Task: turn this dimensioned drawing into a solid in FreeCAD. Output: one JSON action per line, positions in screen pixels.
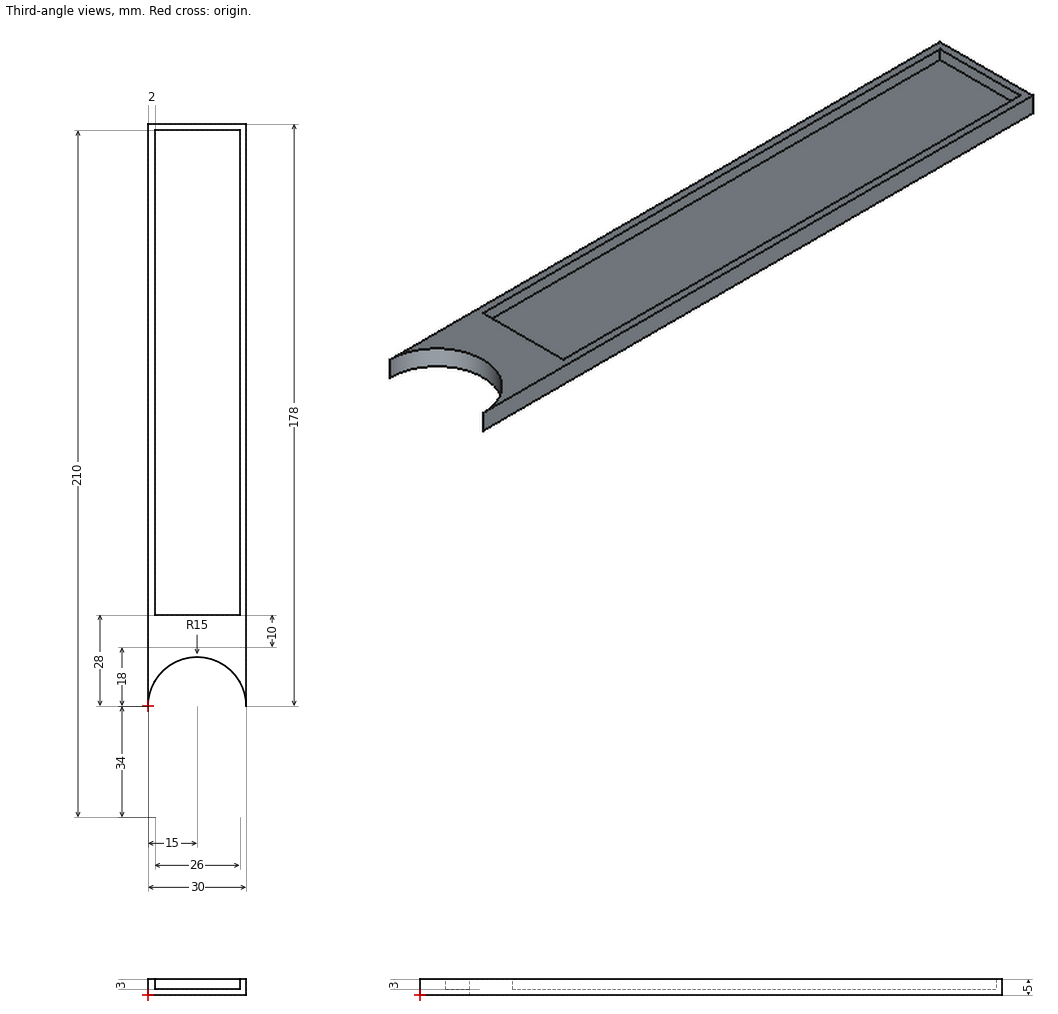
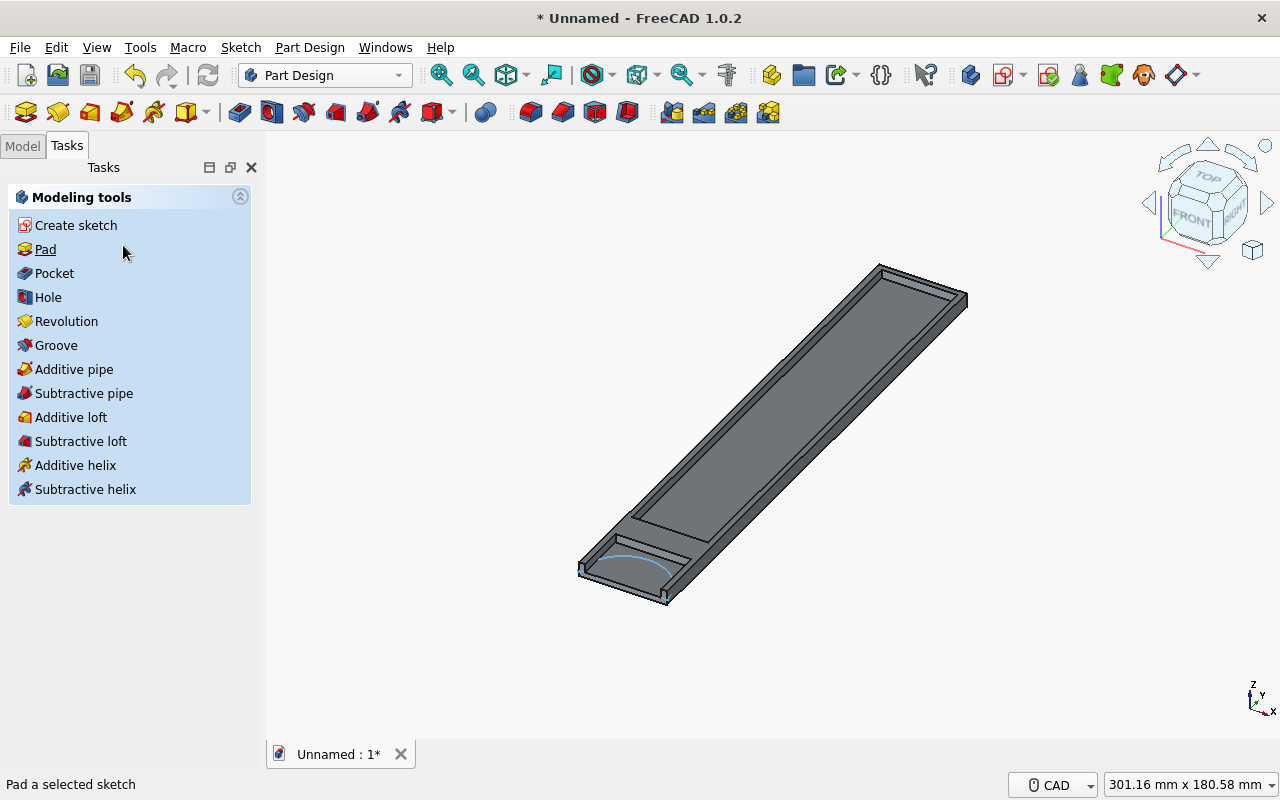
{"action": "left_click", "coordinate": [240, 112]}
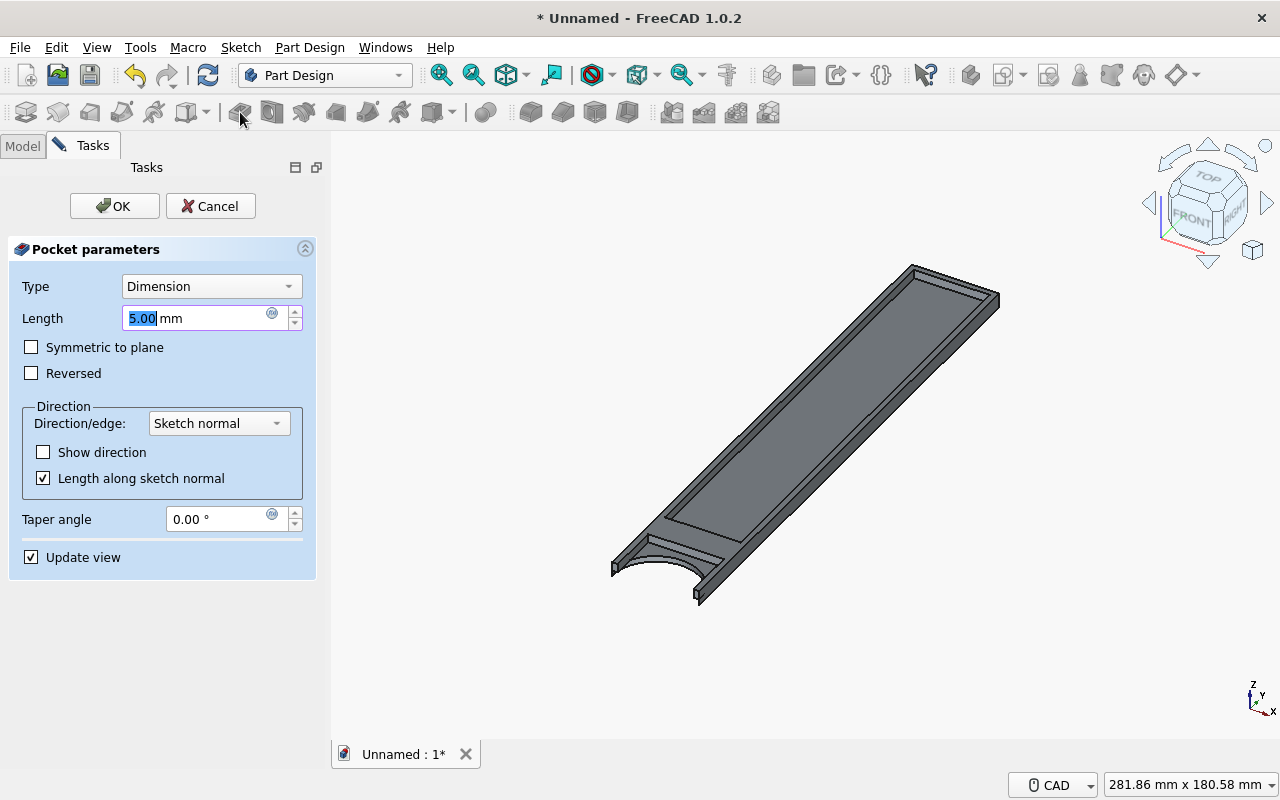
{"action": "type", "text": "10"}
{"action": "key", "text": "Tab"}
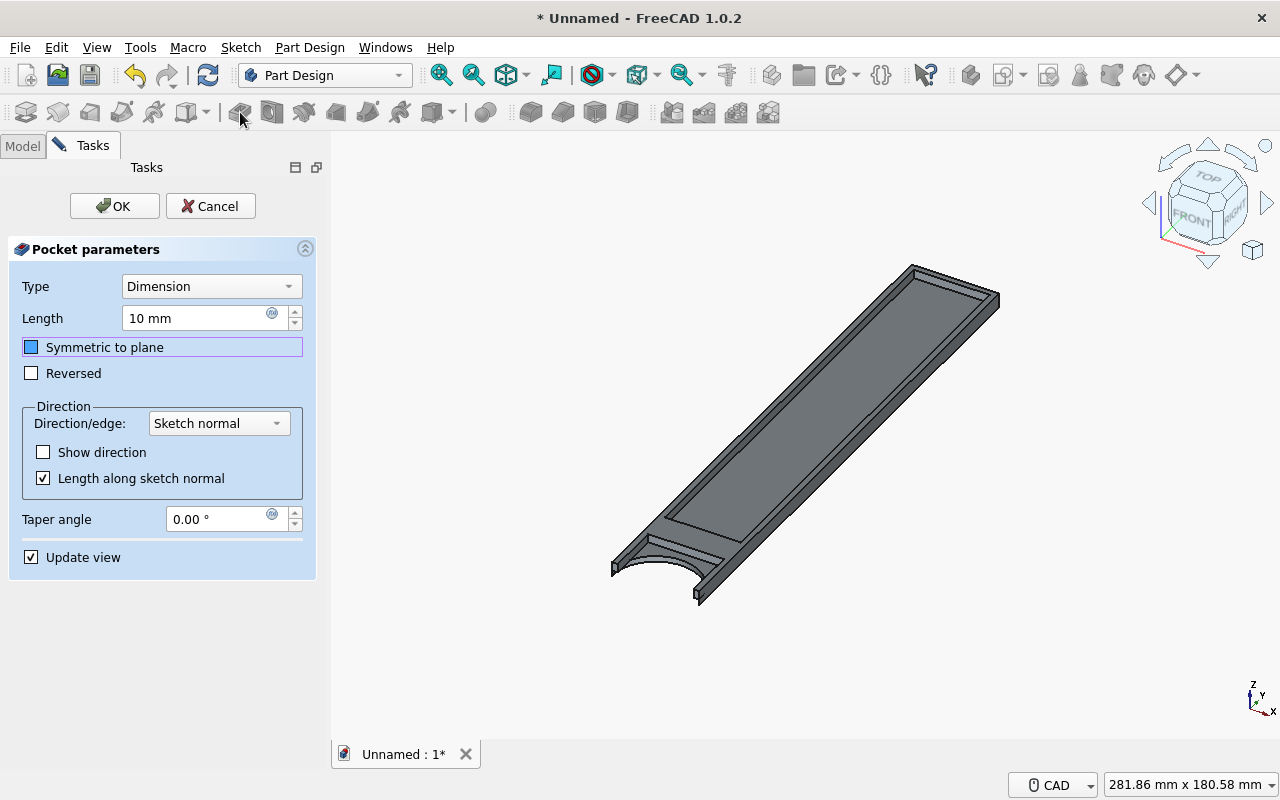
{"action": "left_click", "coordinate": [30, 347]}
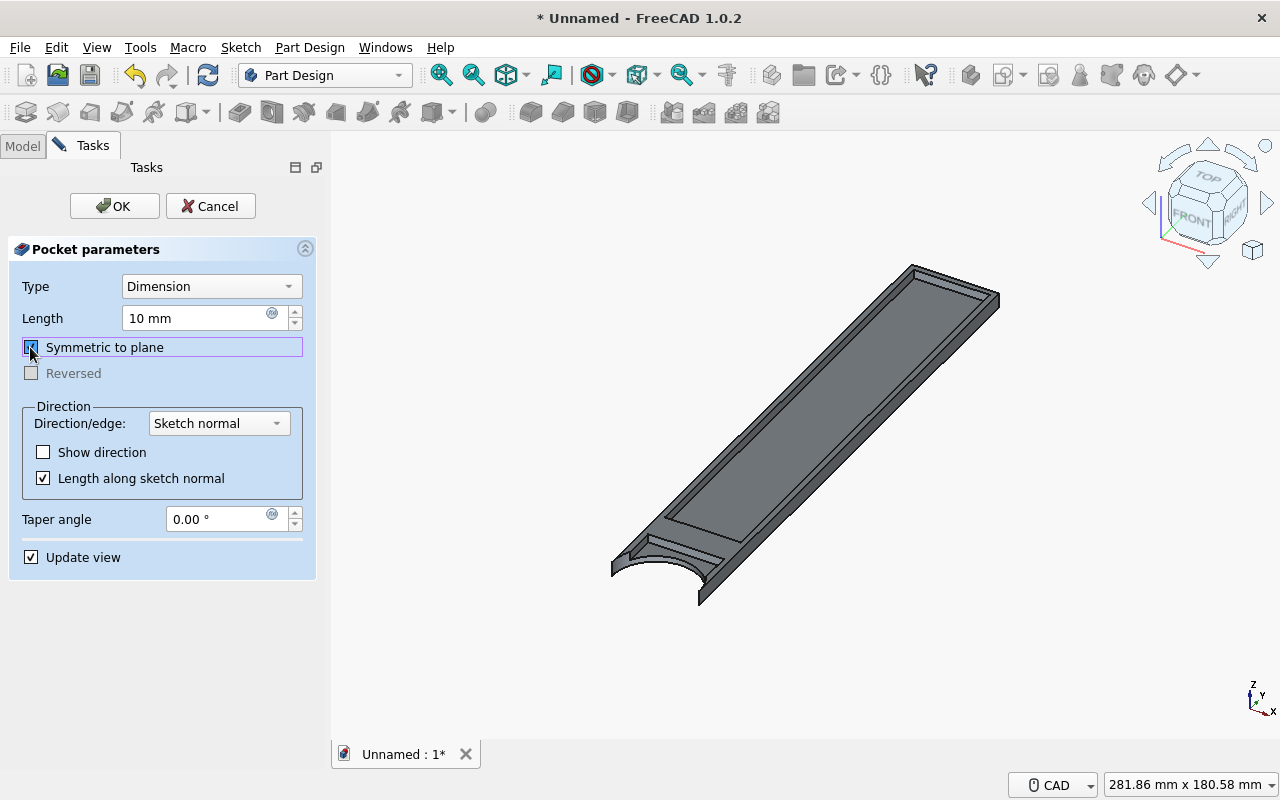
{"action": "left_click", "coordinate": [115, 206]}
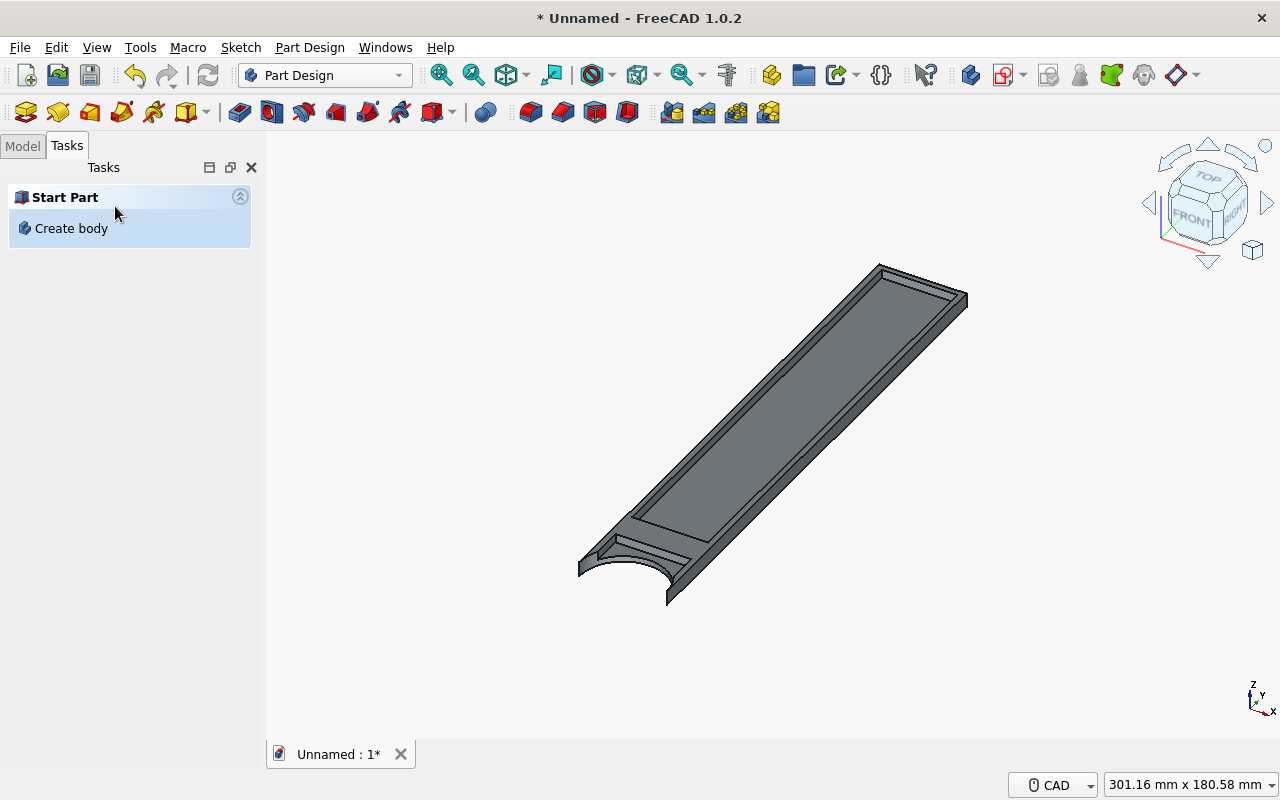
{"action": "left_click", "coordinate": [652, 530]}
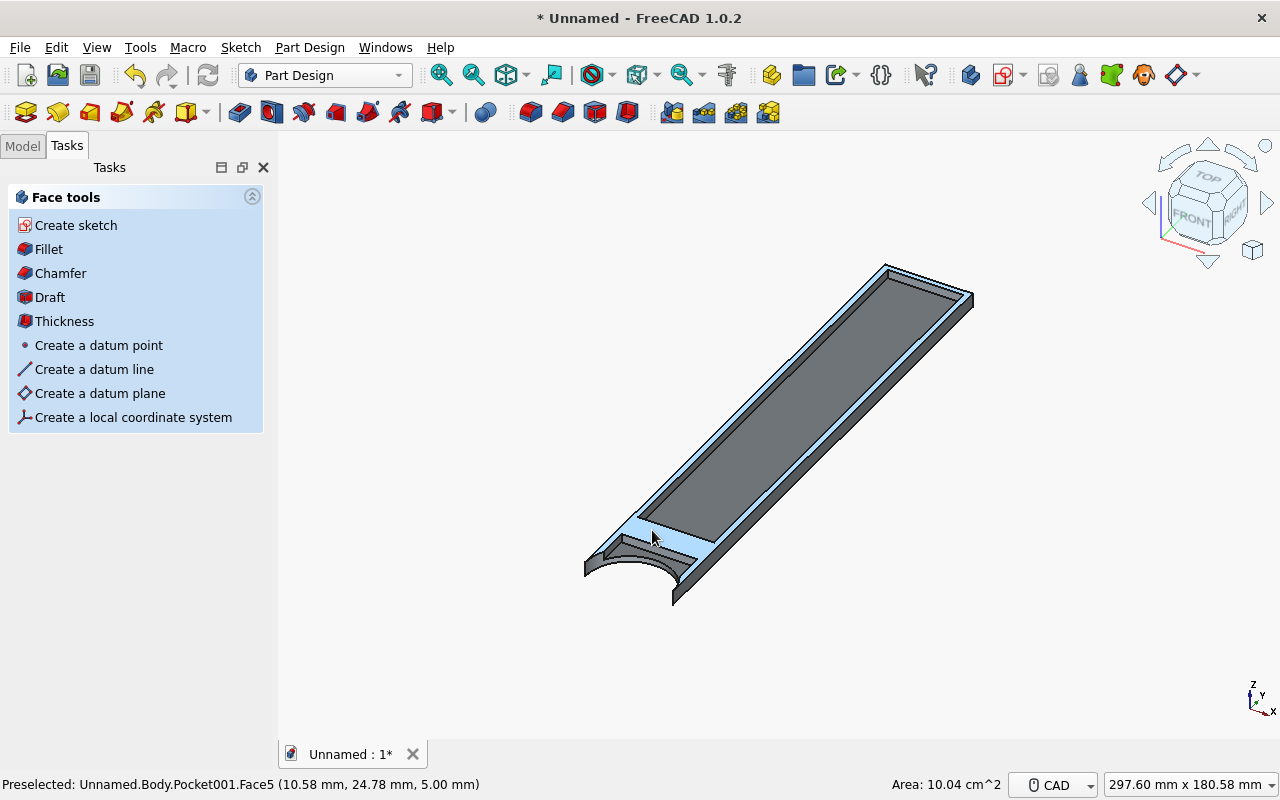
{"action": "left_click", "coordinate": [1004, 76]}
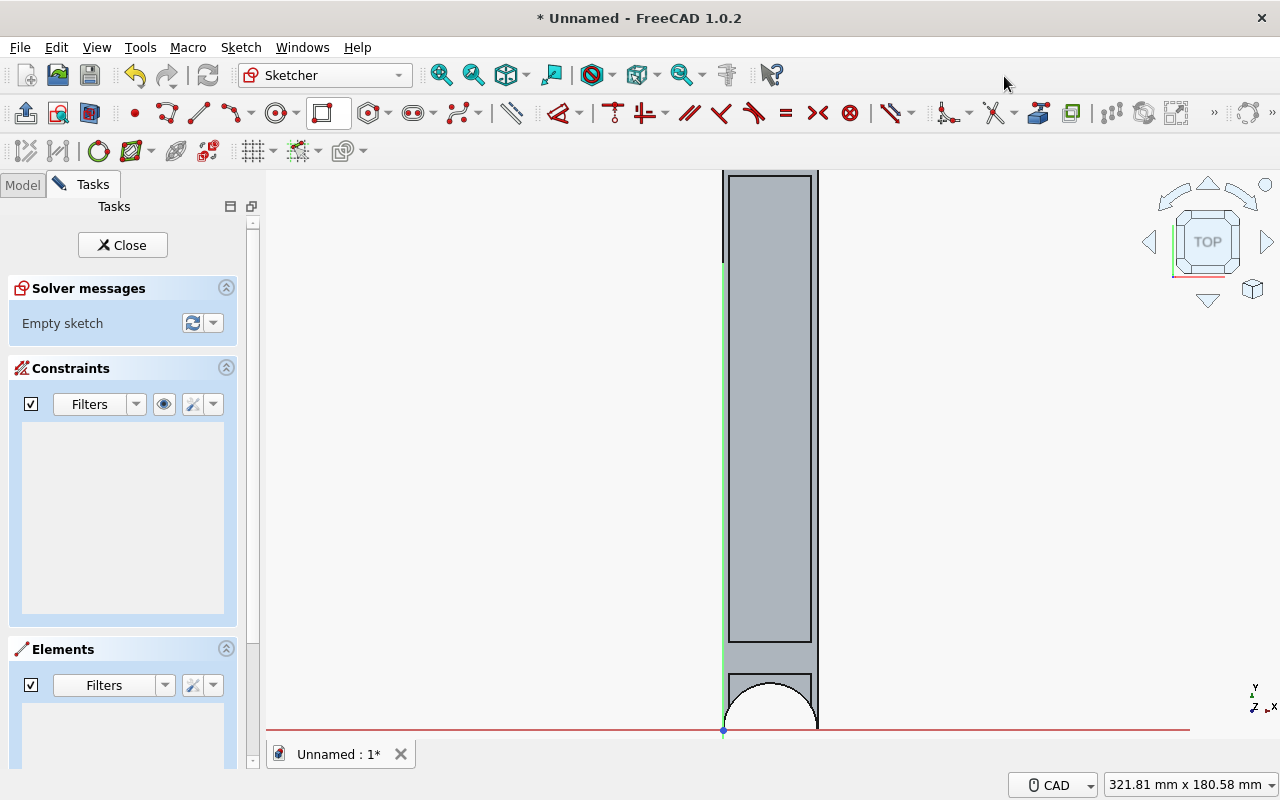
{"action": "scroll", "coordinate": [704, 454], "scroll_direction": "down", "scroll_amount": 5}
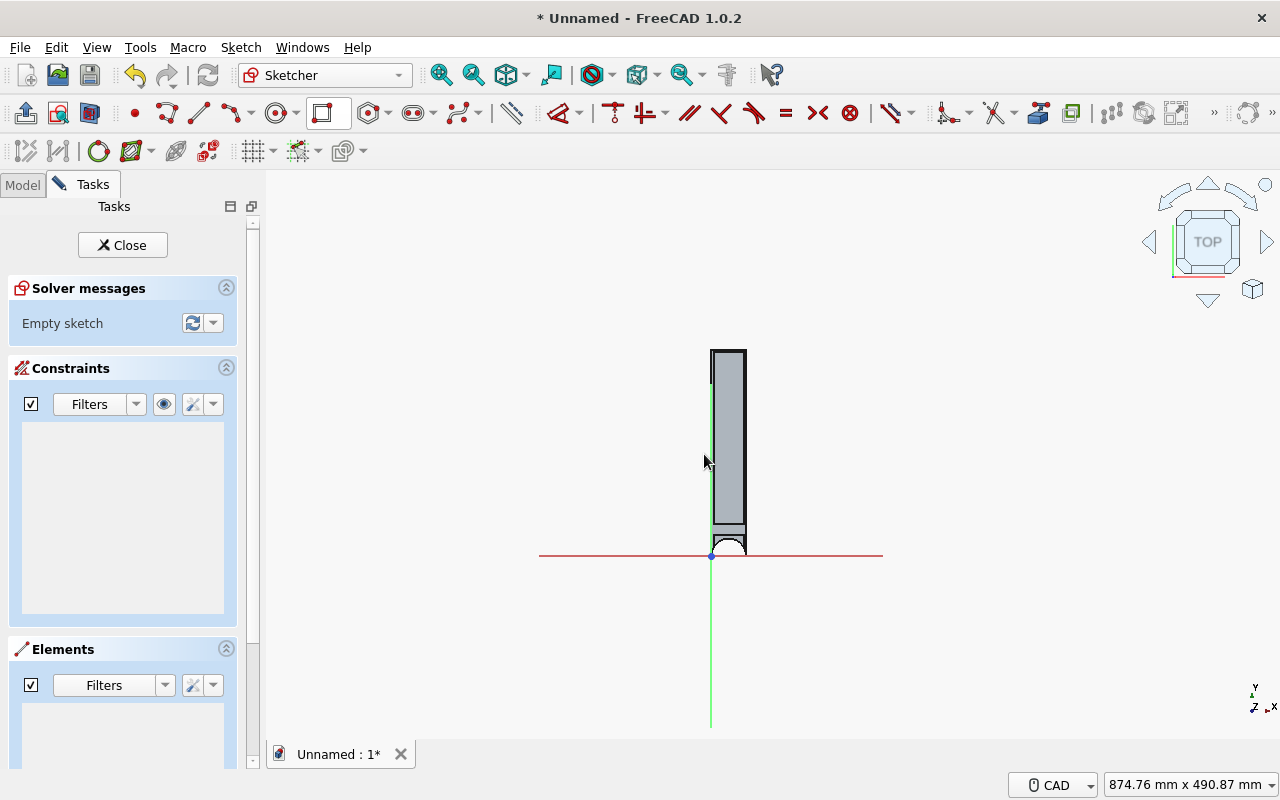
{"action": "scroll", "coordinate": [729, 551], "scroll_direction": "up", "scroll_amount": 14}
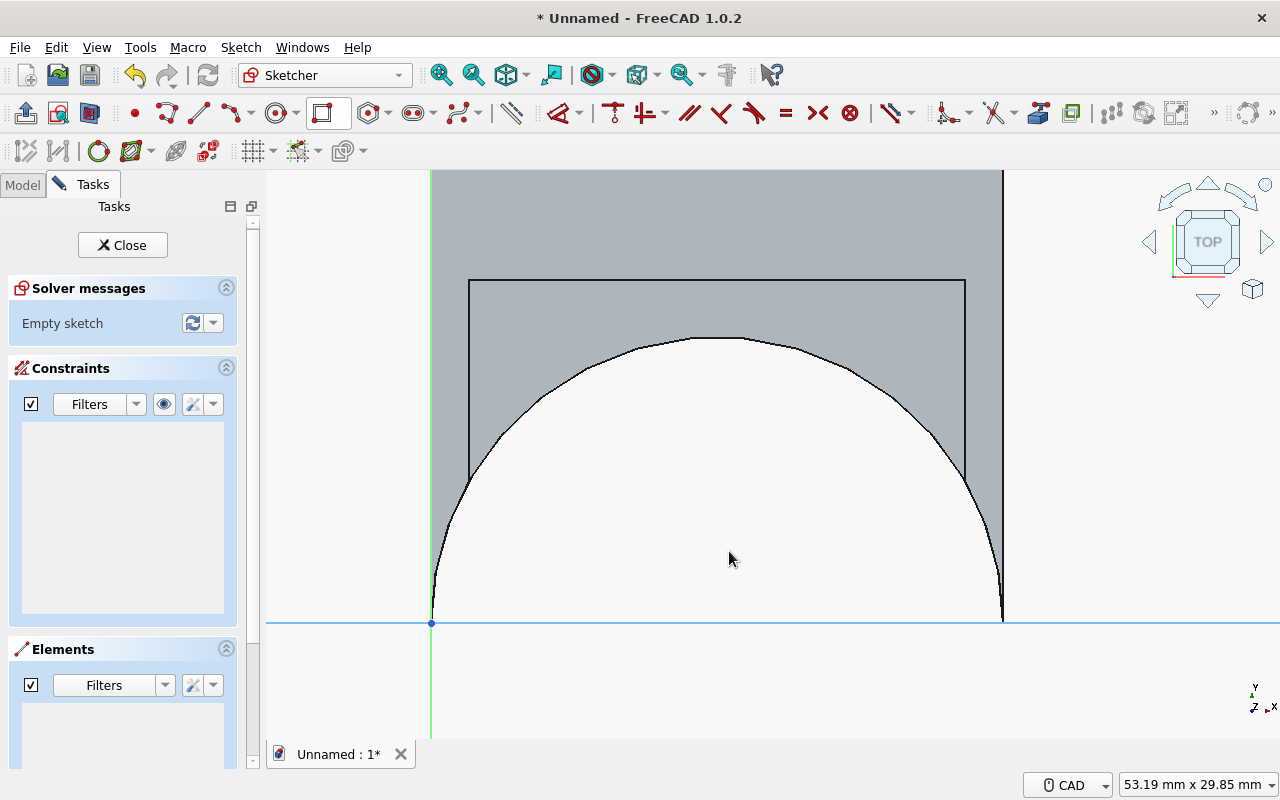
{"action": "left_click", "coordinate": [168, 114]}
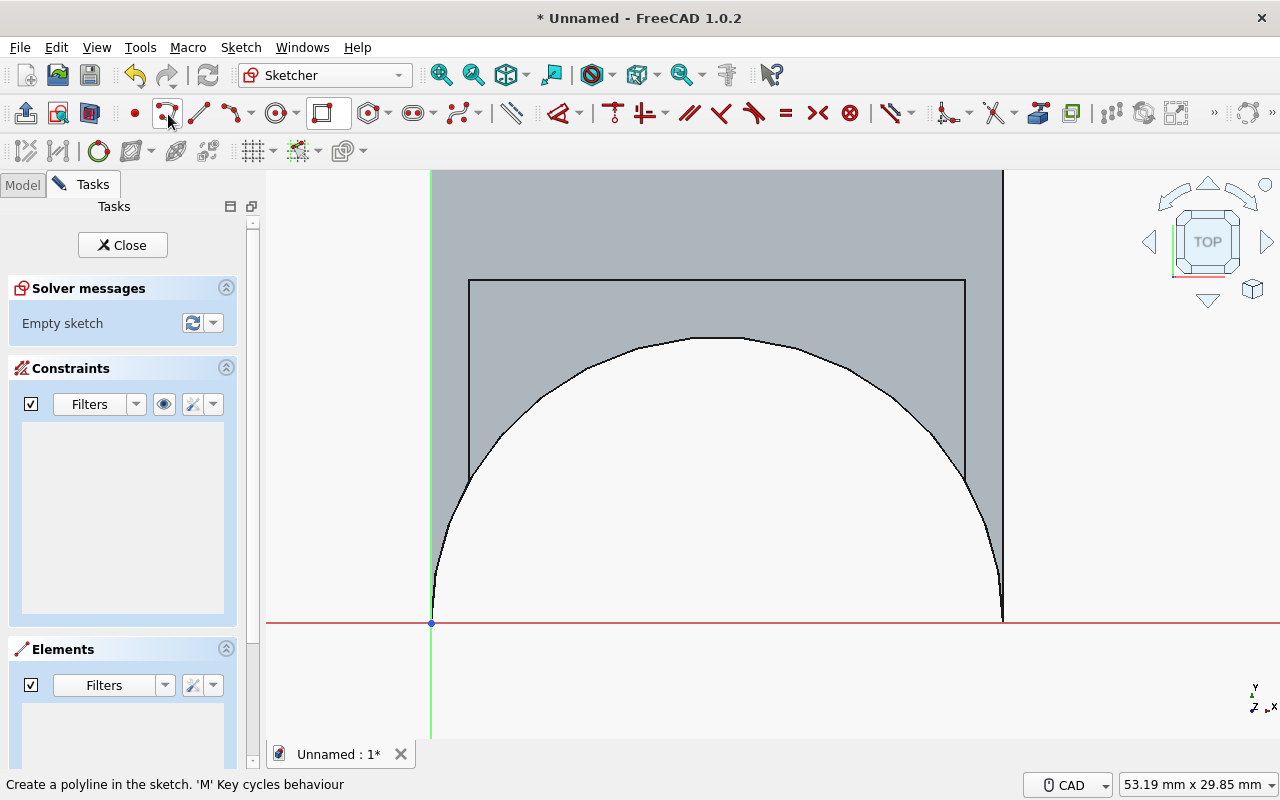
{"action": "left_click", "coordinate": [965, 480]}
{"action": "left_click", "coordinate": [965, 280]}
{"action": "left_click", "coordinate": [469, 280]}
{"action": "left_click", "coordinate": [469, 480]}
{"action": "right_click", "coordinate": [469, 480]}